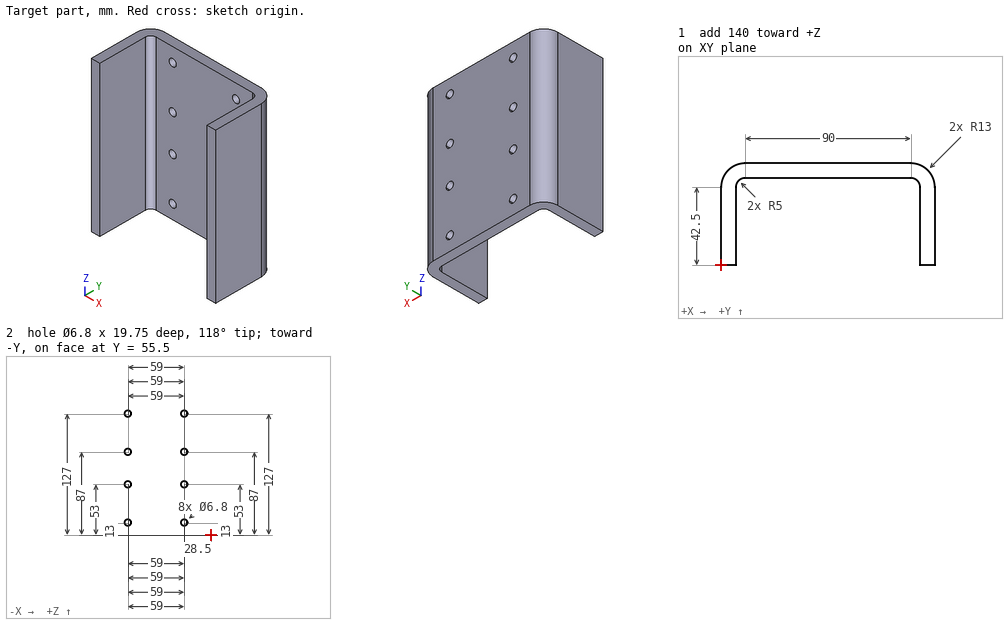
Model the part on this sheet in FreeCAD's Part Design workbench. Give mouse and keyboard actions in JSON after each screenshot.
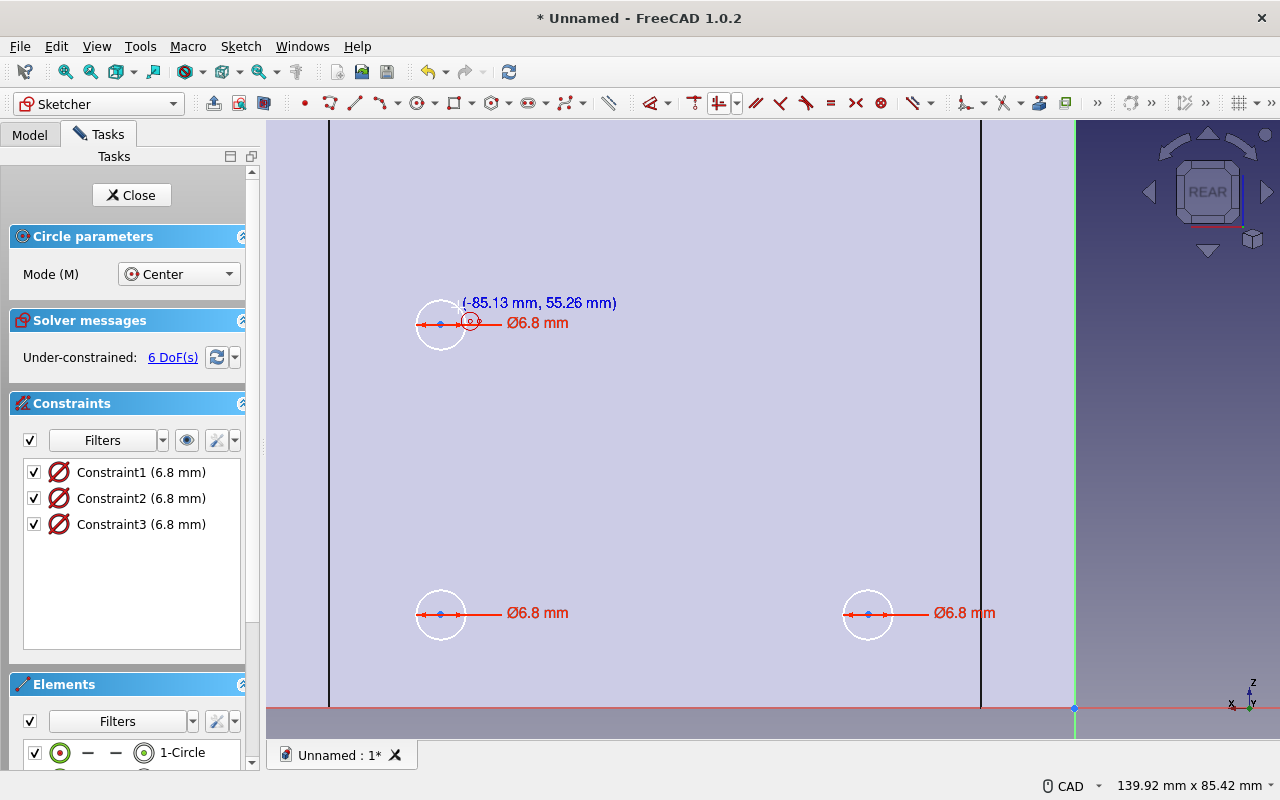
{"action": "left_click", "coordinate": [868, 324]}
{"action": "mouse_move", "coordinate": [886, 307]}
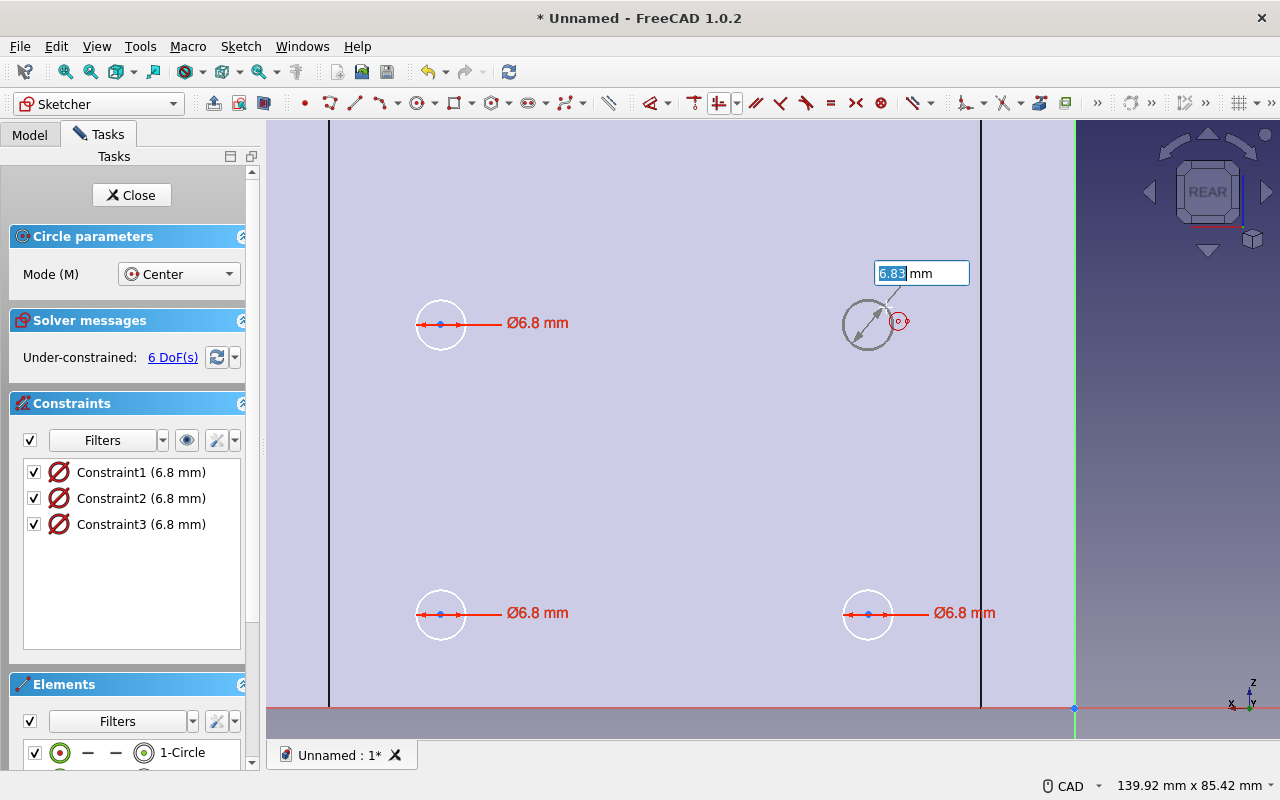
{"action": "type", "text": "6.8"}
{"action": "key", "text": "Return"}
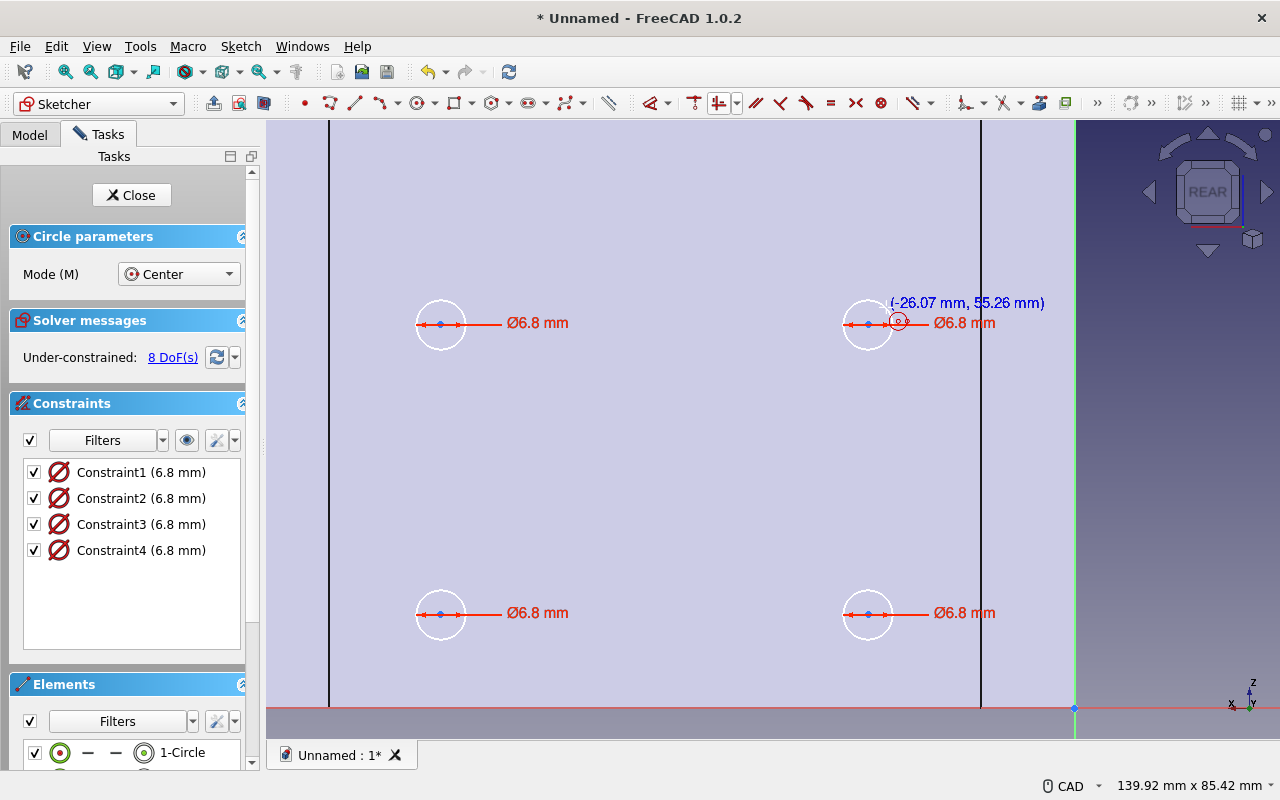
{"action": "scroll", "coordinate": [671, 587], "scroll_direction": "down", "scroll_amount": 4}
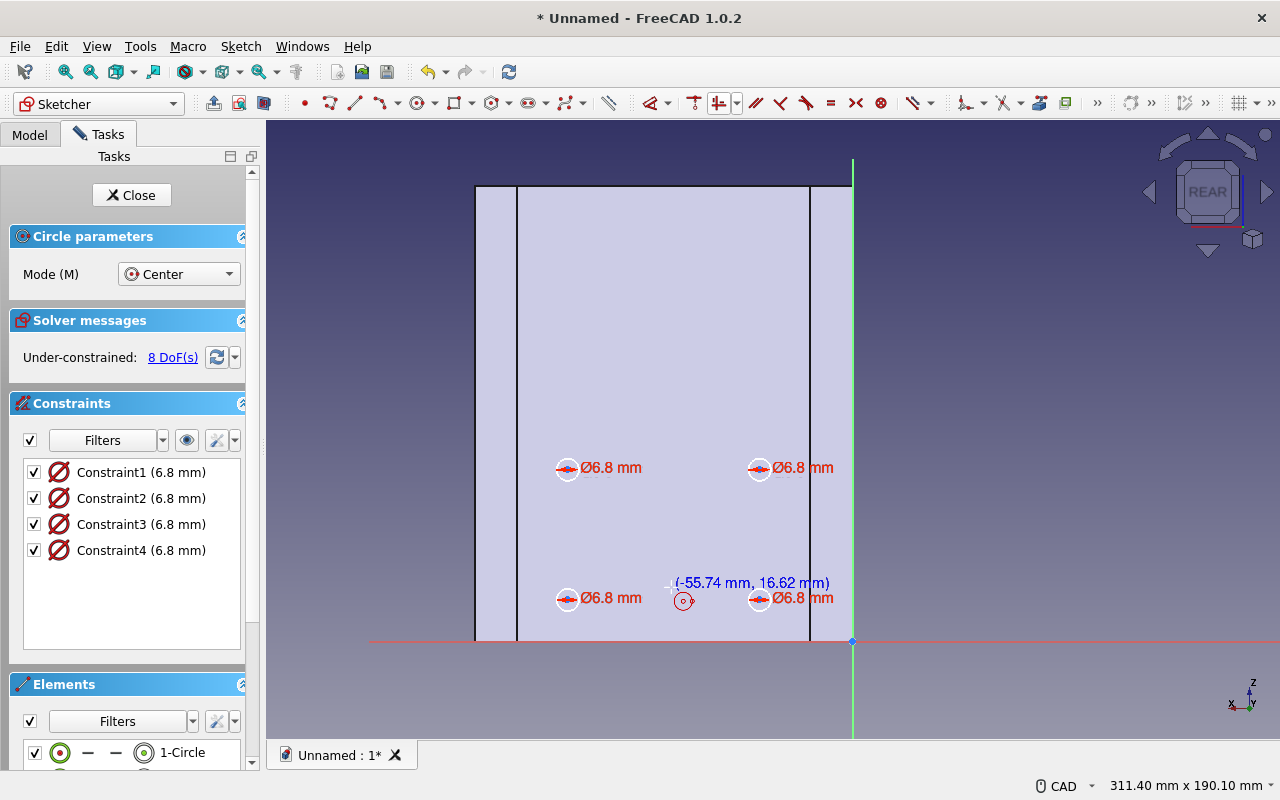
{"action": "scroll", "coordinate": [760, 359], "scroll_direction": "up", "scroll_amount": 4}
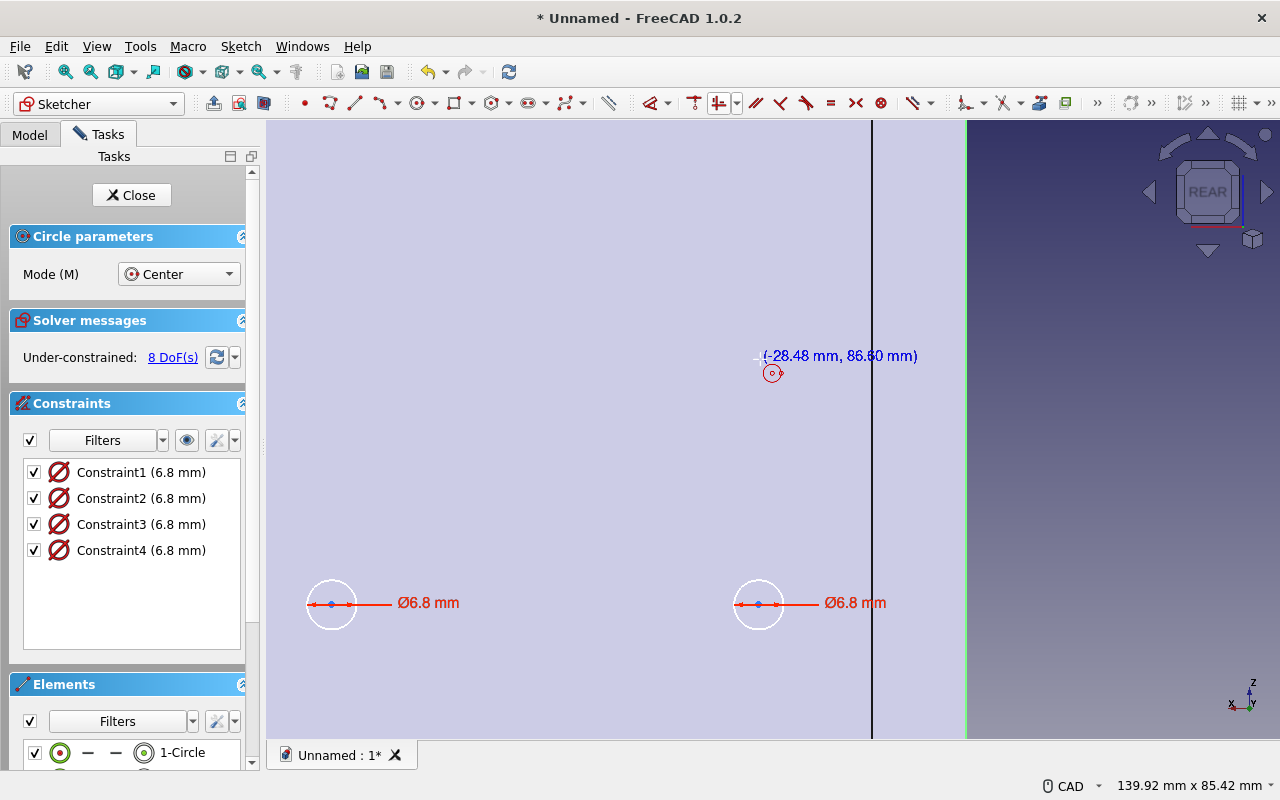
{"action": "left_click", "coordinate": [759, 358]}
{"action": "mouse_move", "coordinate": [777, 340]}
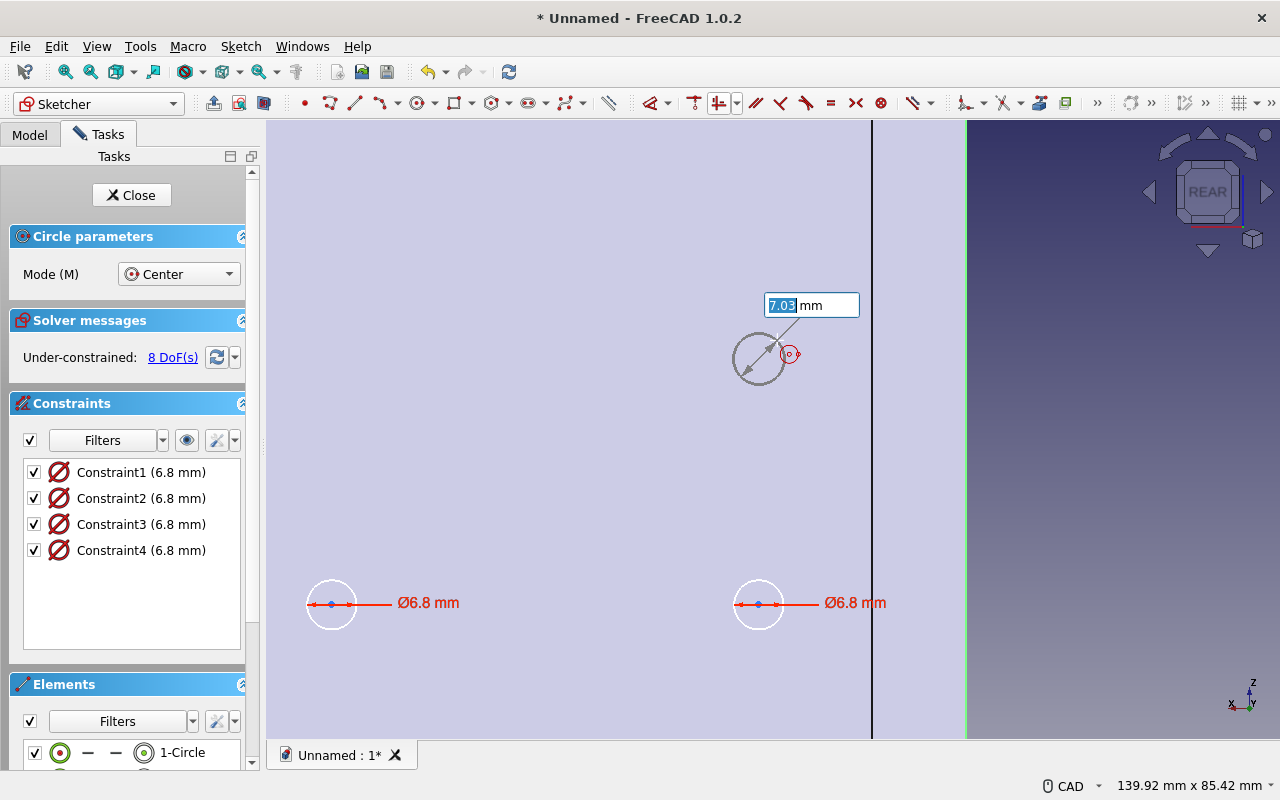
{"action": "type", "text": "6.8"}
{"action": "key", "text": "Return"}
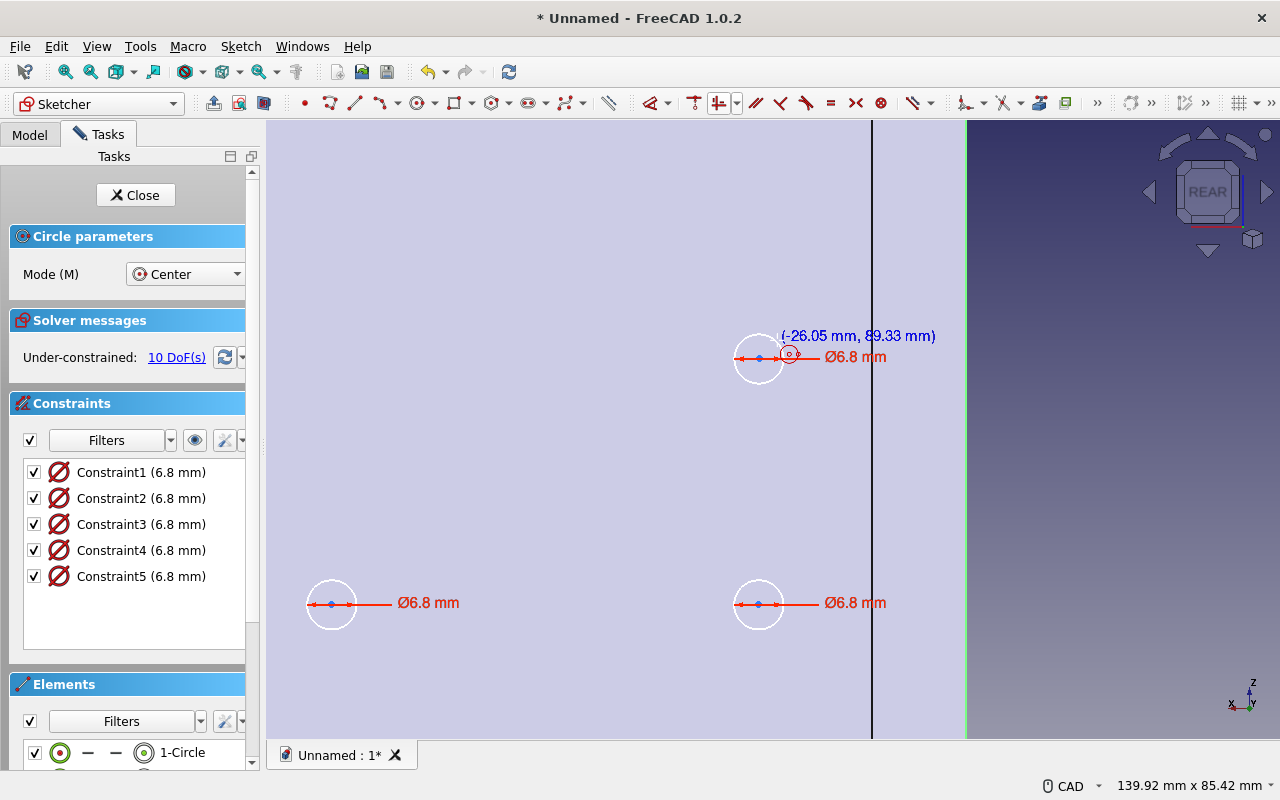
{"action": "left_click", "coordinate": [332, 358]}
{"action": "mouse_move", "coordinate": [349, 340]}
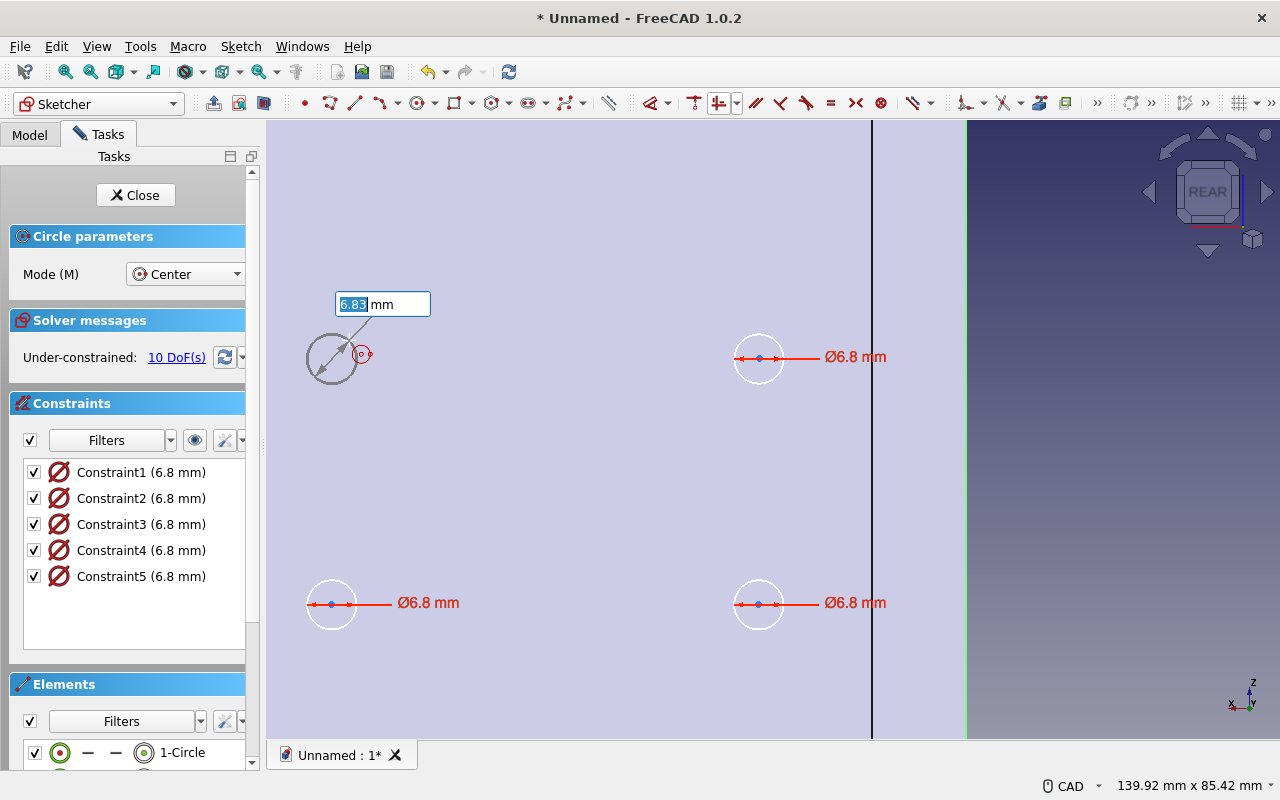
{"action": "type", "text": "6.8"}
{"action": "key", "text": "Return"}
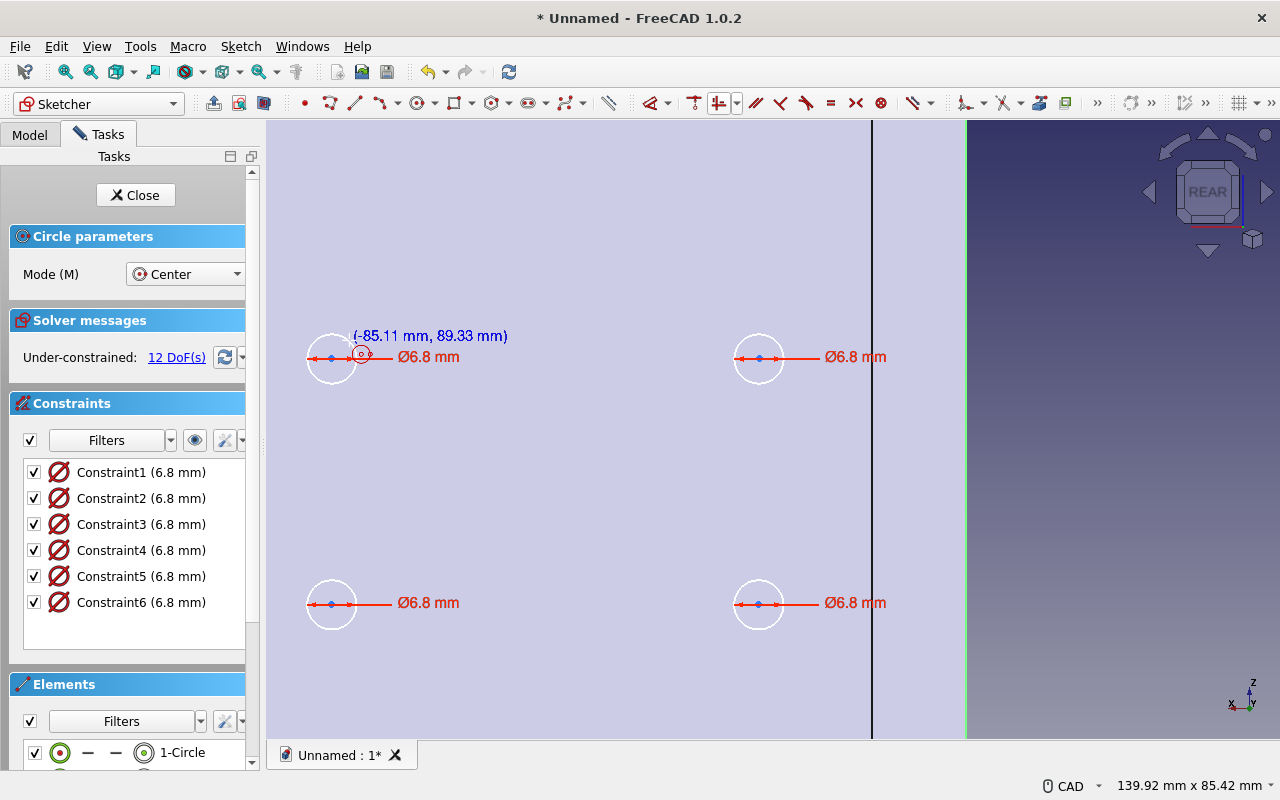
{"action": "scroll", "coordinate": [760, 359], "scroll_direction": "down", "scroll_amount": 4}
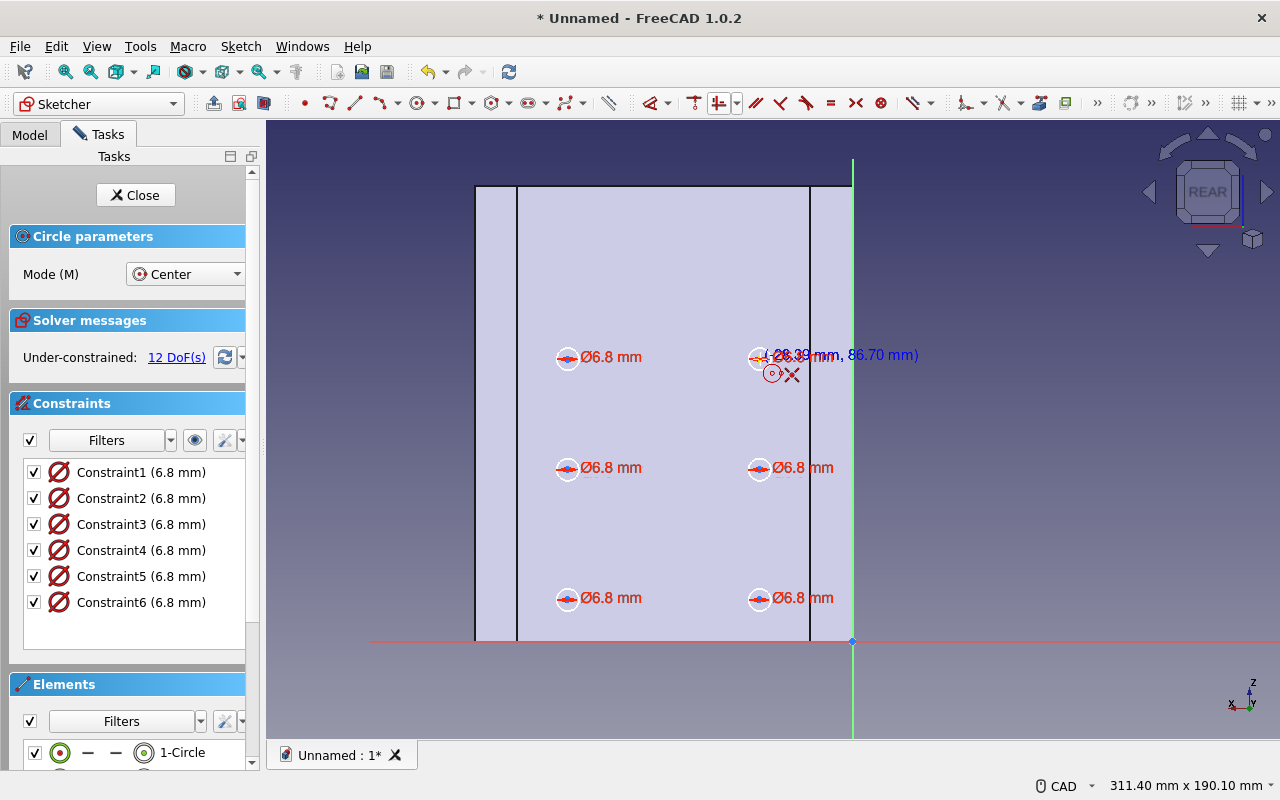
{"action": "scroll", "coordinate": [568, 228], "scroll_direction": "up", "scroll_amount": 4}